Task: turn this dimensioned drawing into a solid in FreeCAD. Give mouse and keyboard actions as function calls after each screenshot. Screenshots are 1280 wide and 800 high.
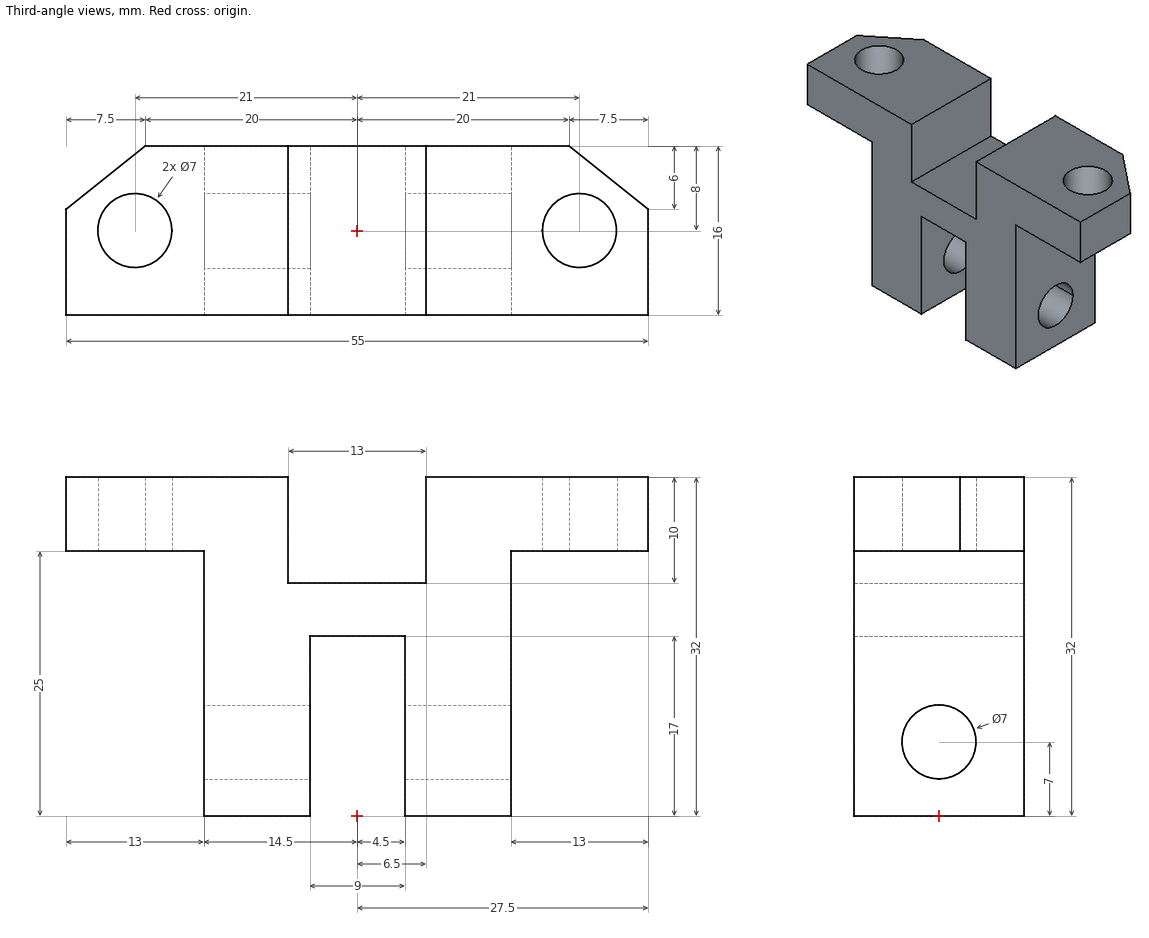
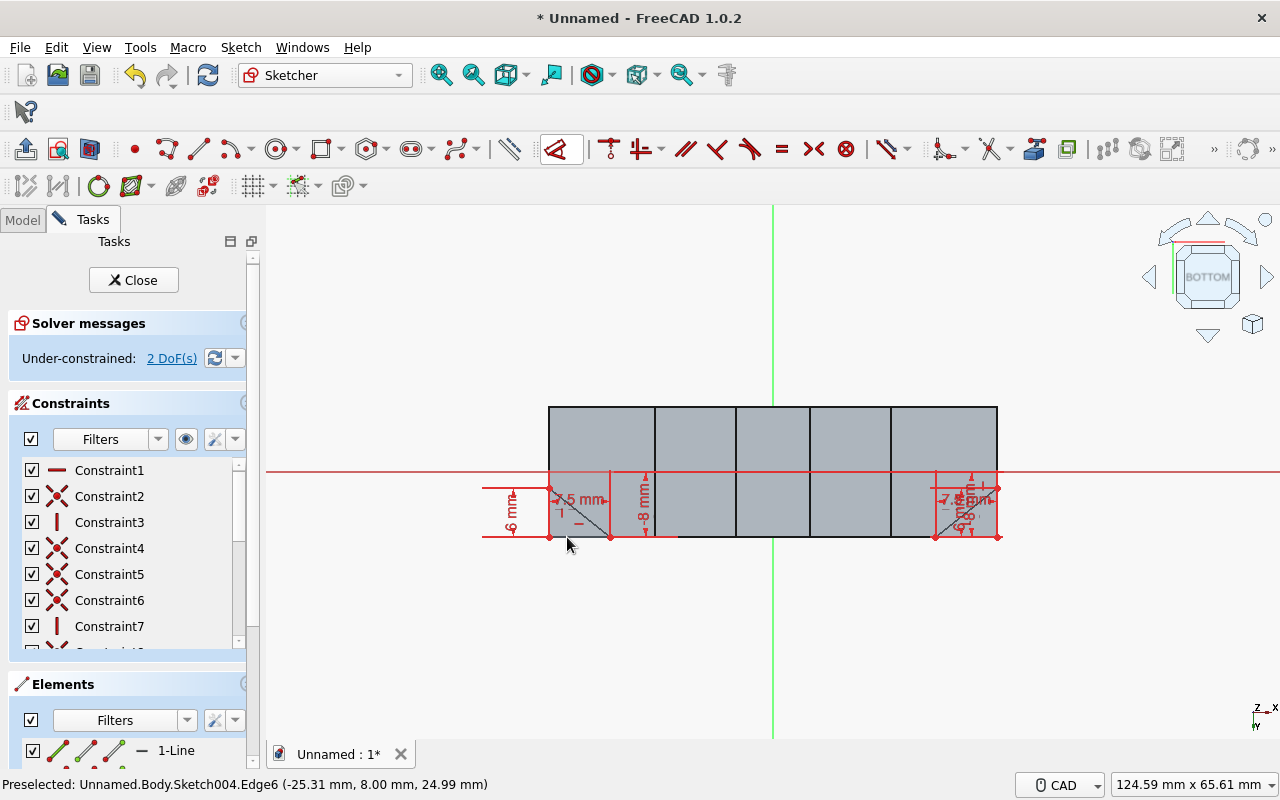
click(936, 537)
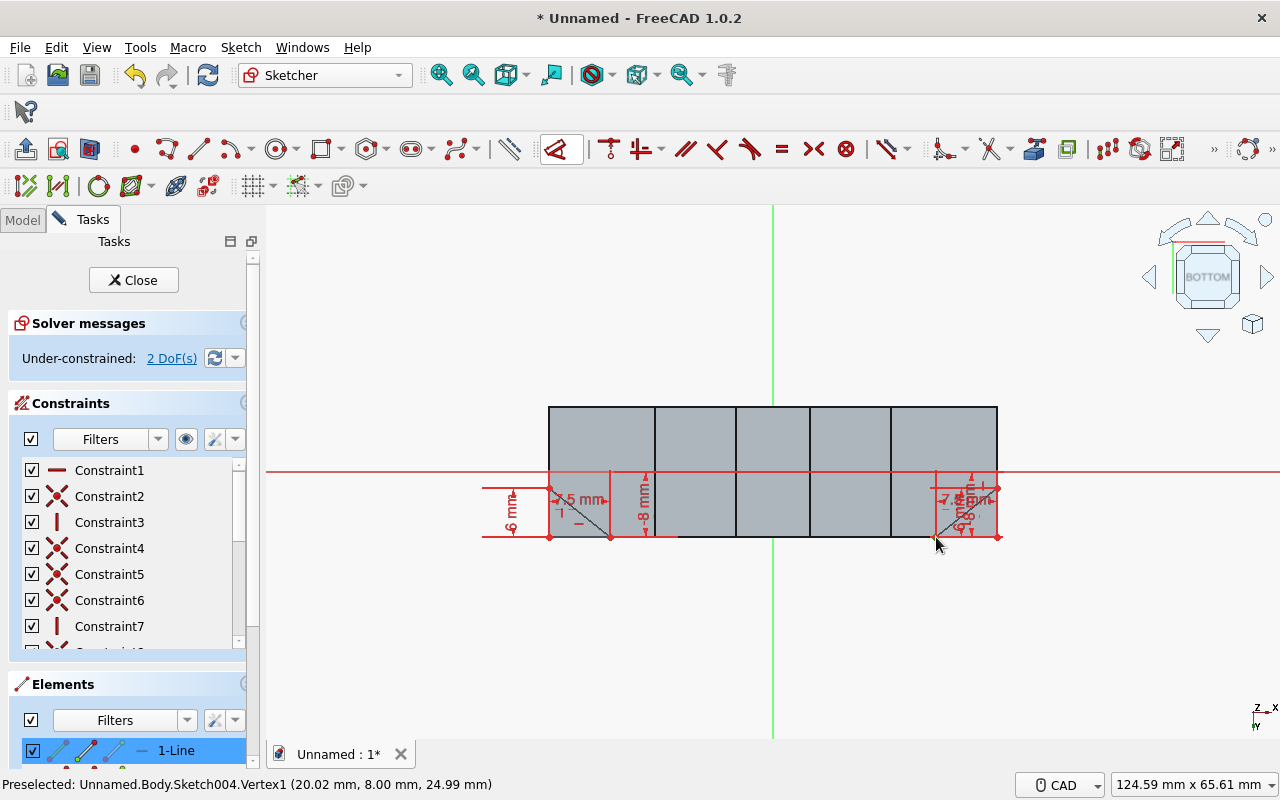
key(l)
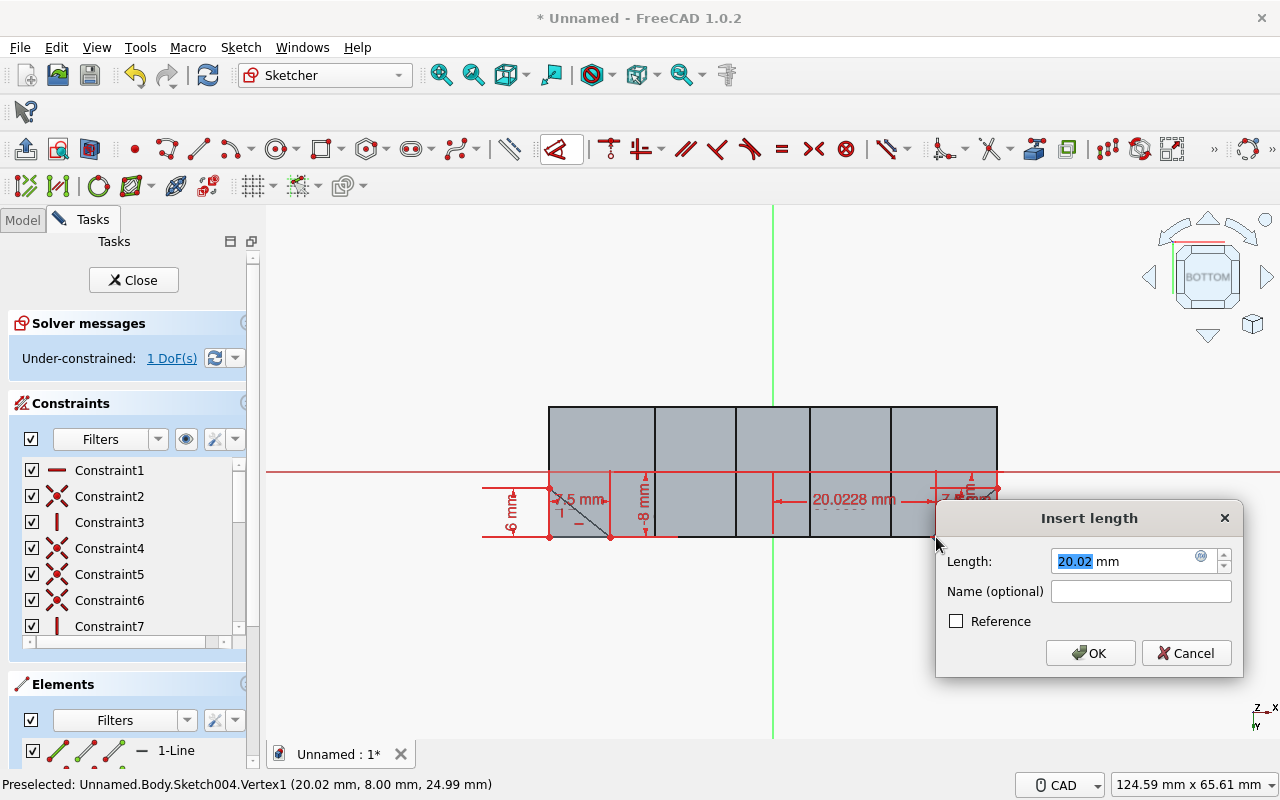
text(20)
key(Return)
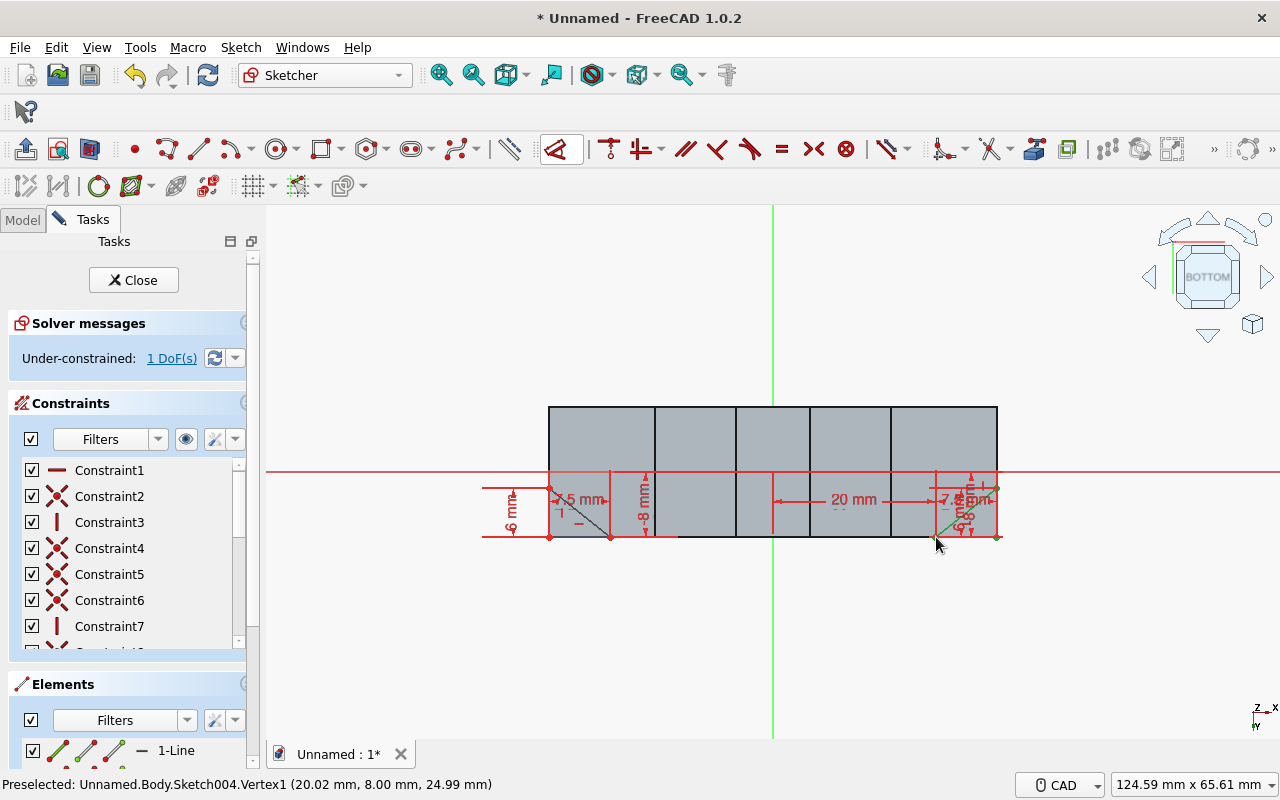
click(610, 537)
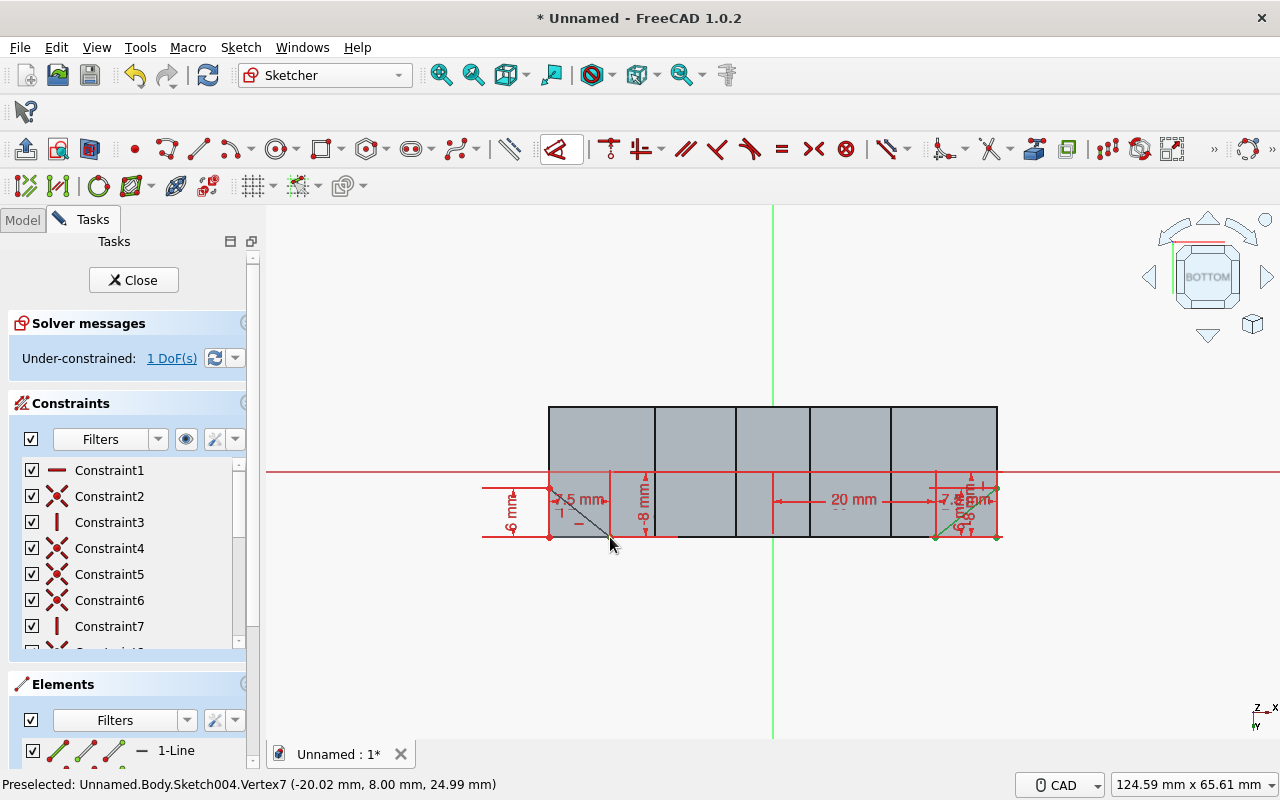
click(578, 150)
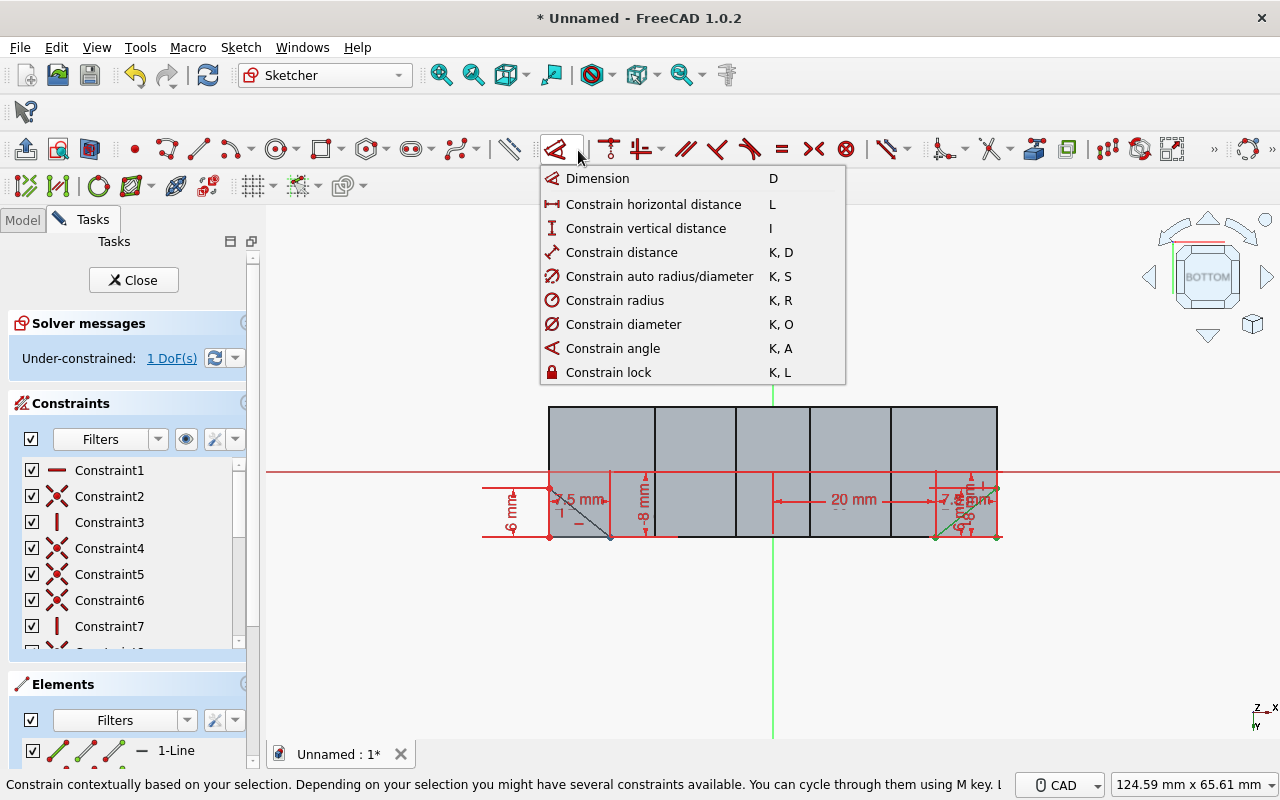
click(693, 204)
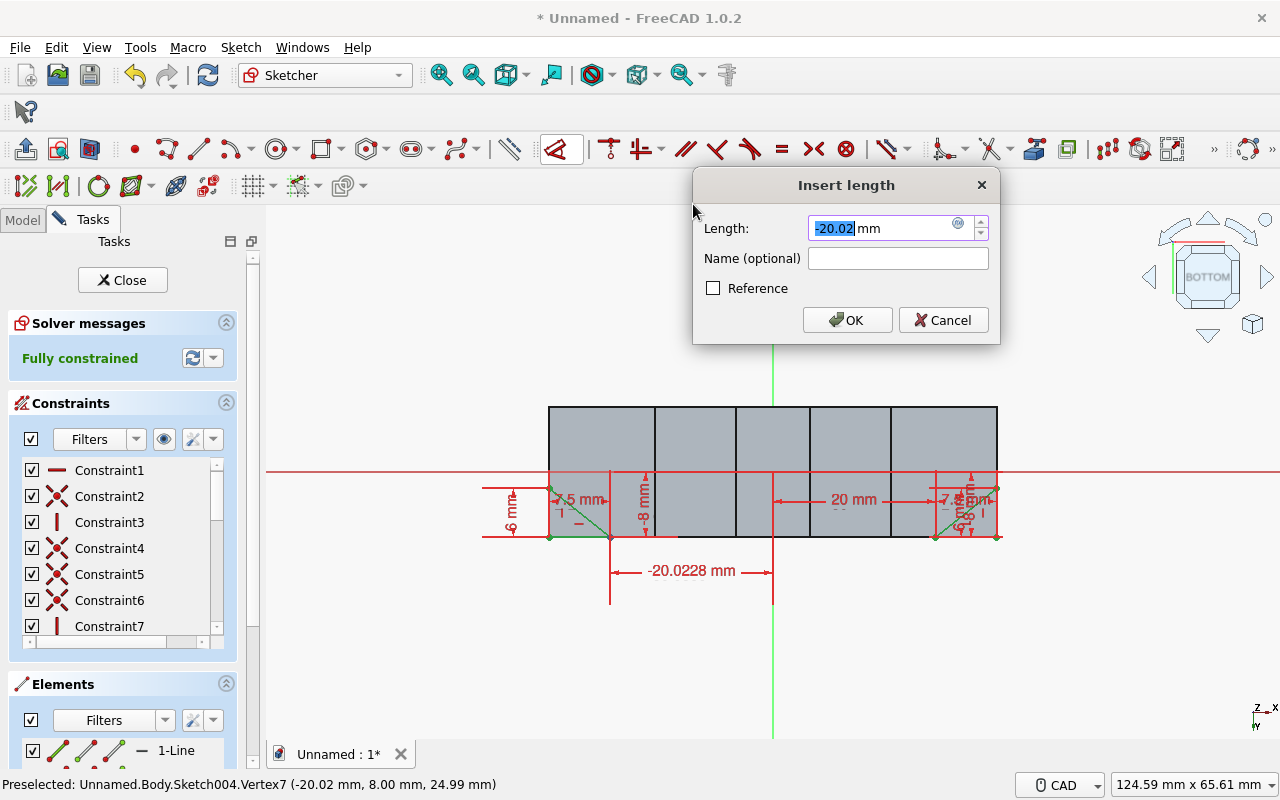
text(-20)
key(Return)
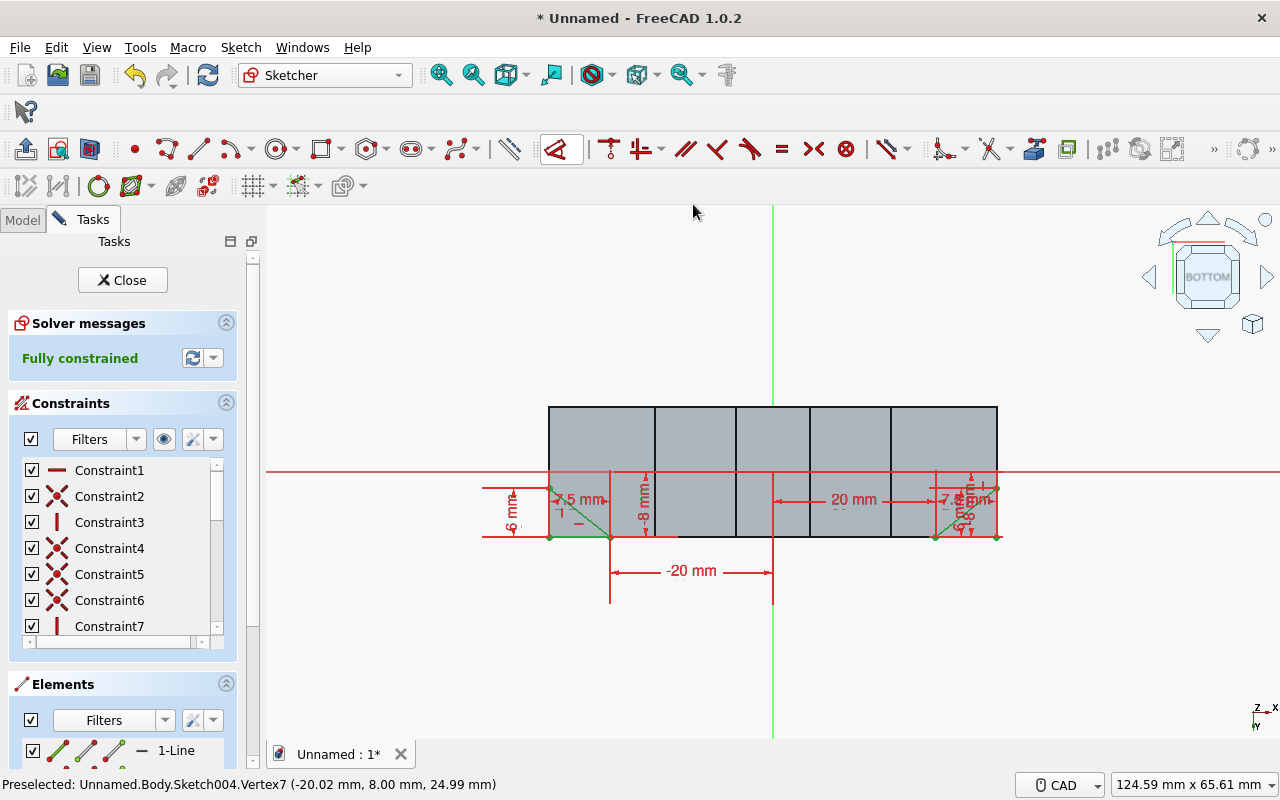
click(123, 280)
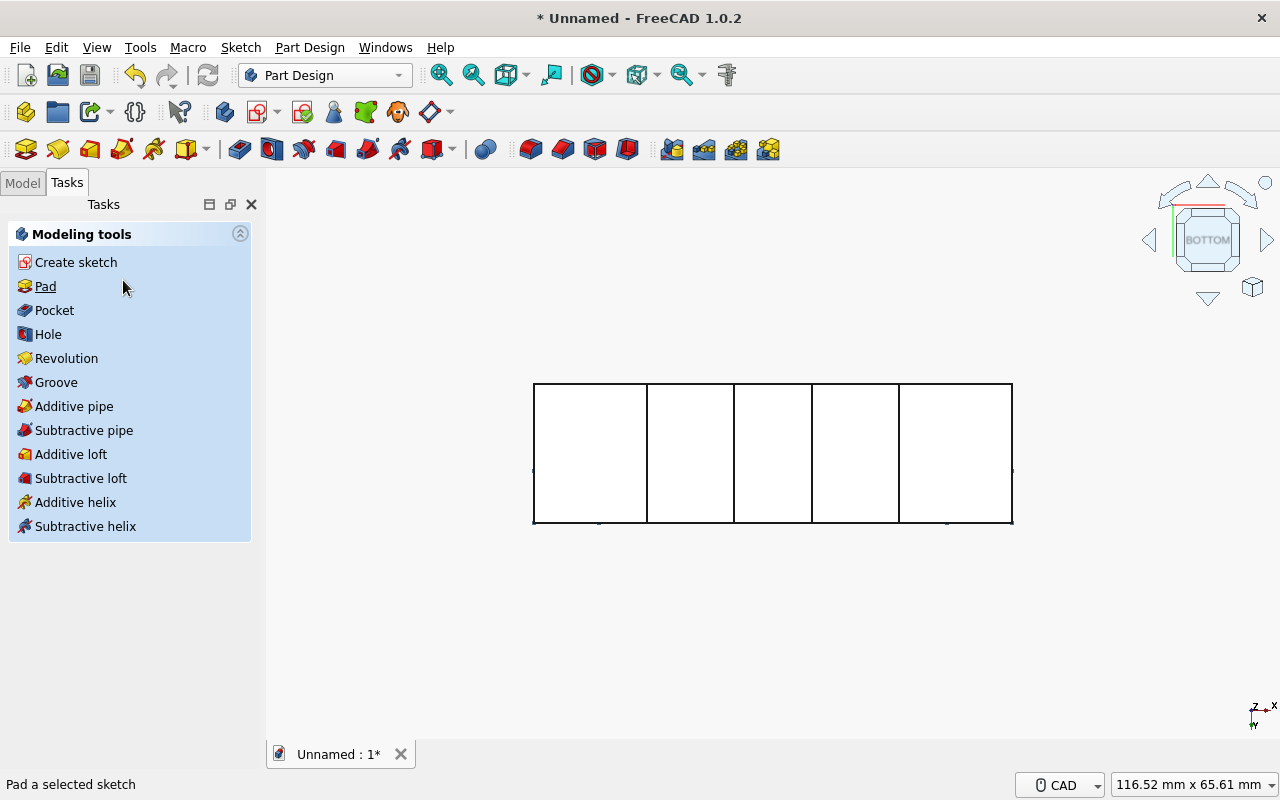
click(240, 150)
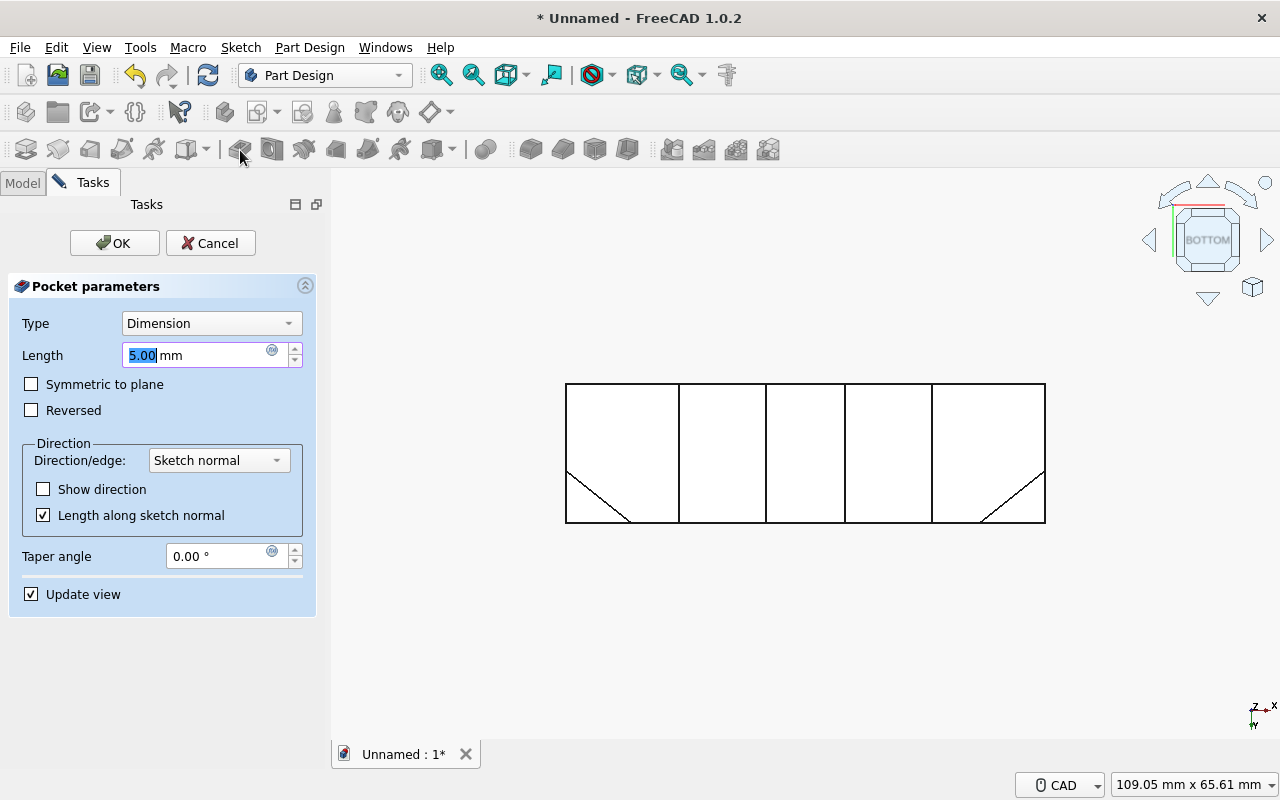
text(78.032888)
key(Tab)